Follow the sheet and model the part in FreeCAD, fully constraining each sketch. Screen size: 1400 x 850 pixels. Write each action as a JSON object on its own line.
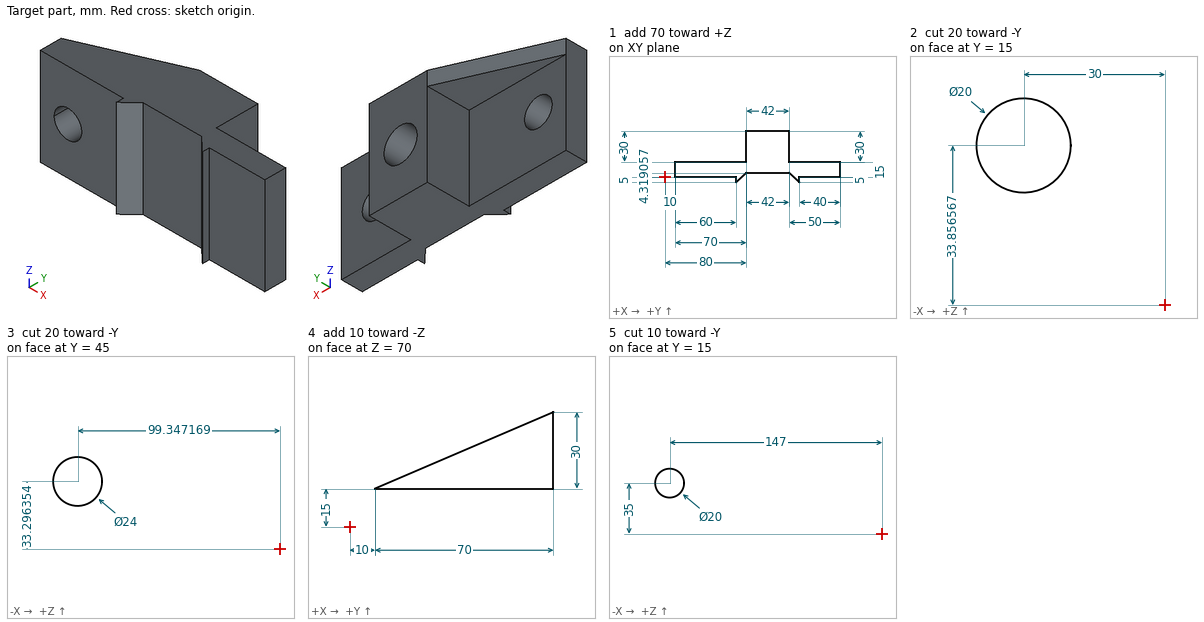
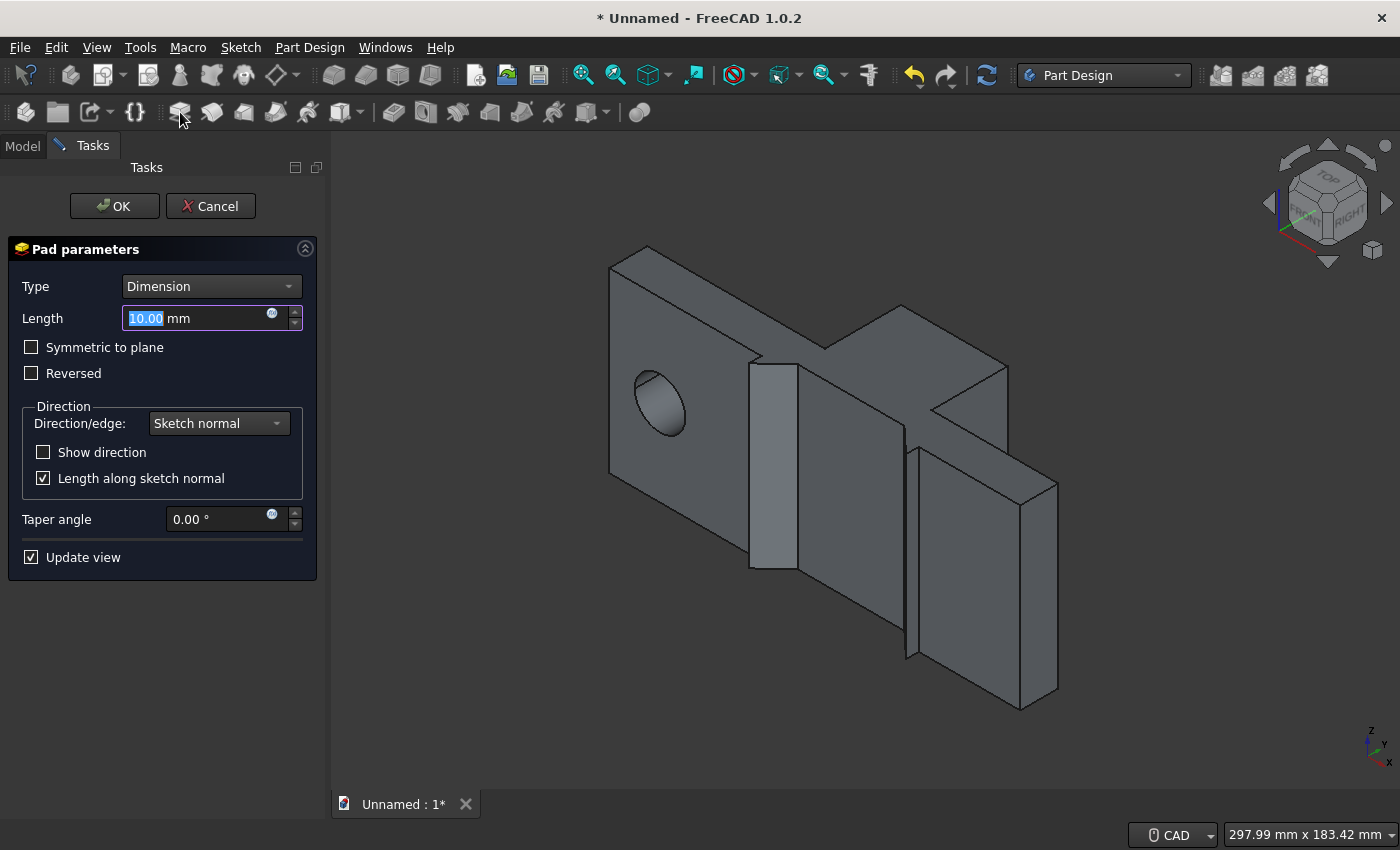
{"action": "type", "text": "10"}
{"action": "key", "text": "Tab"}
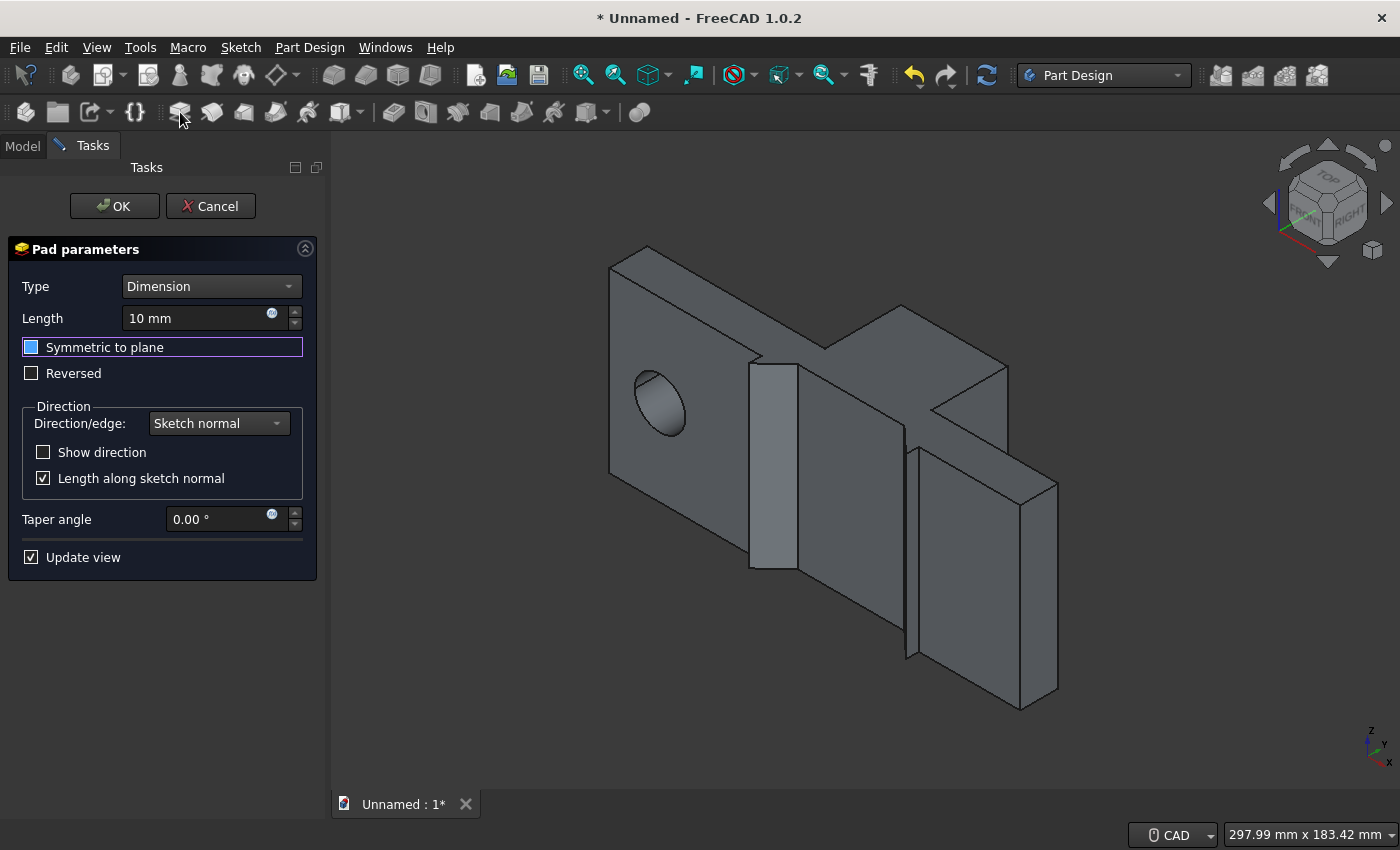
{"action": "left_click", "coordinate": [30, 373]}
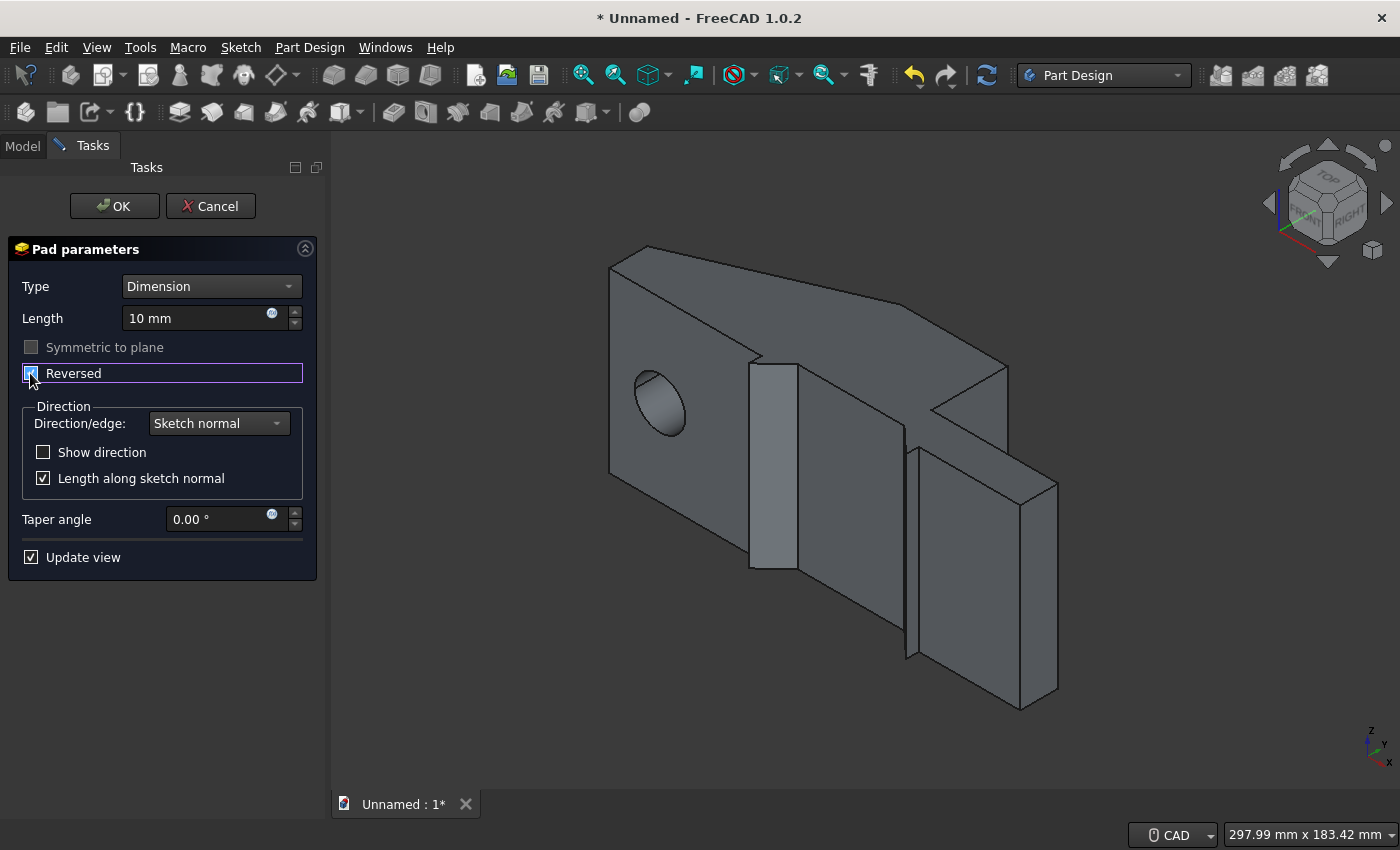
{"action": "left_click", "coordinate": [115, 206]}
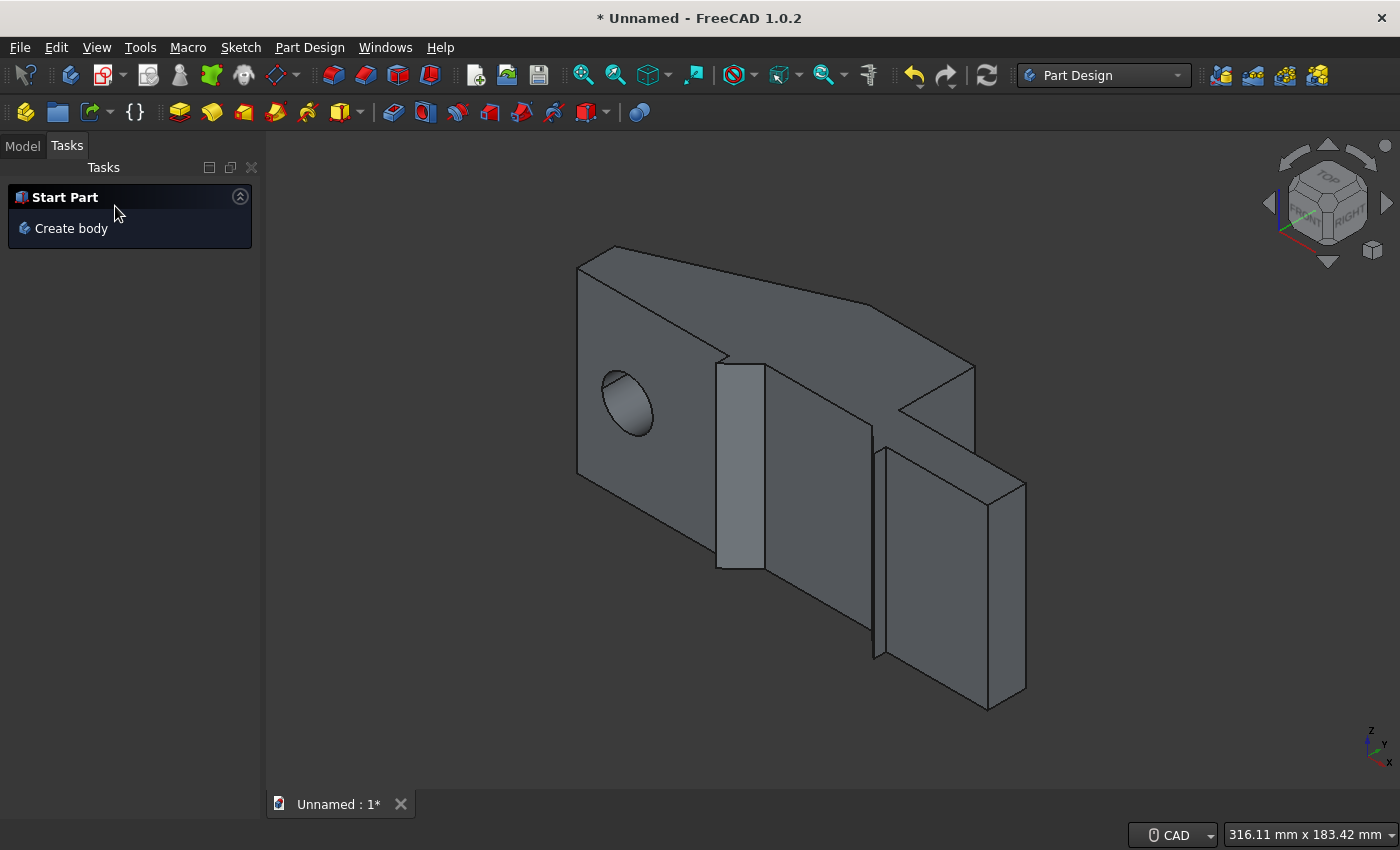
{"action": "key", "text": "4"}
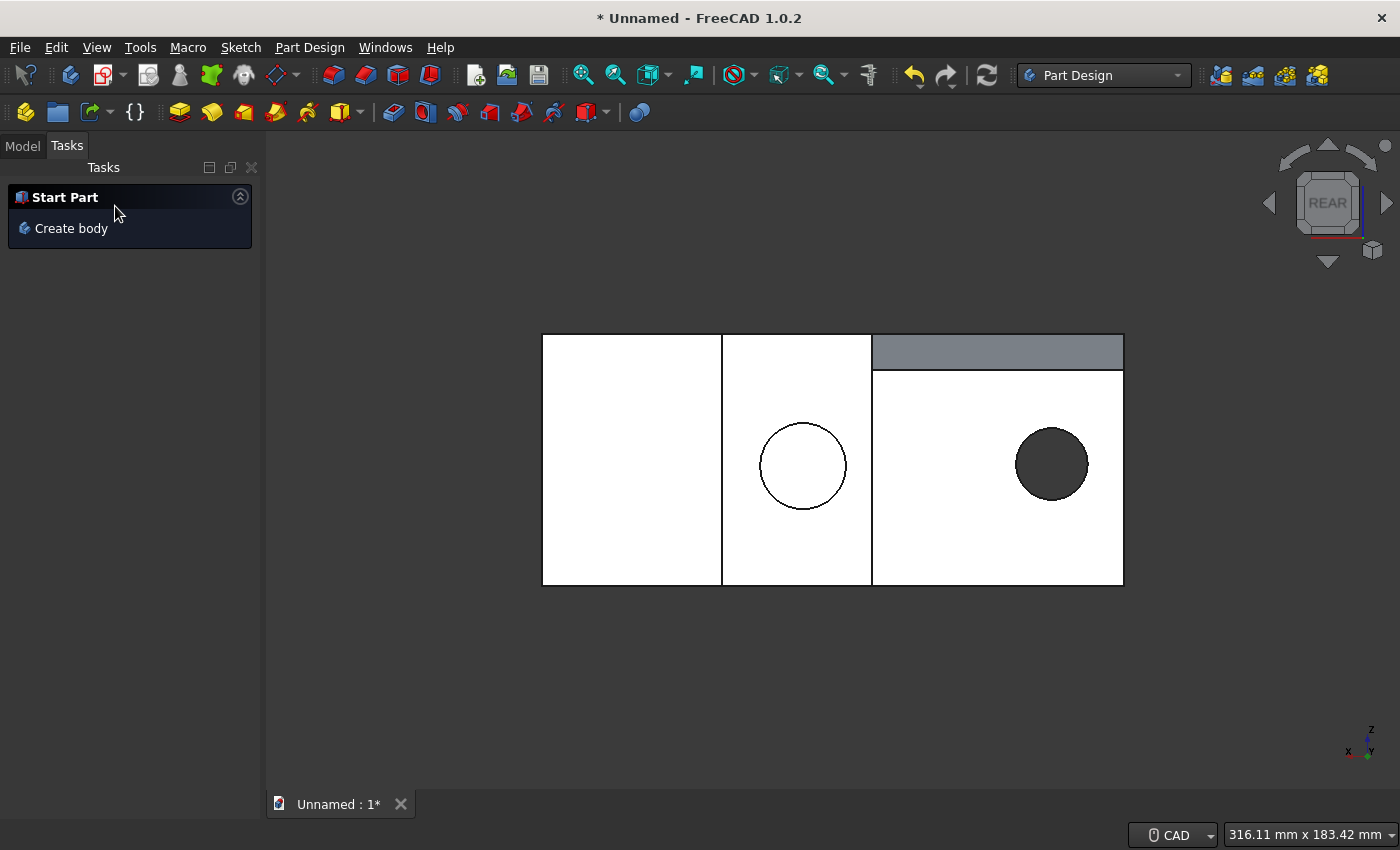
{"action": "left_click", "coordinate": [962, 508]}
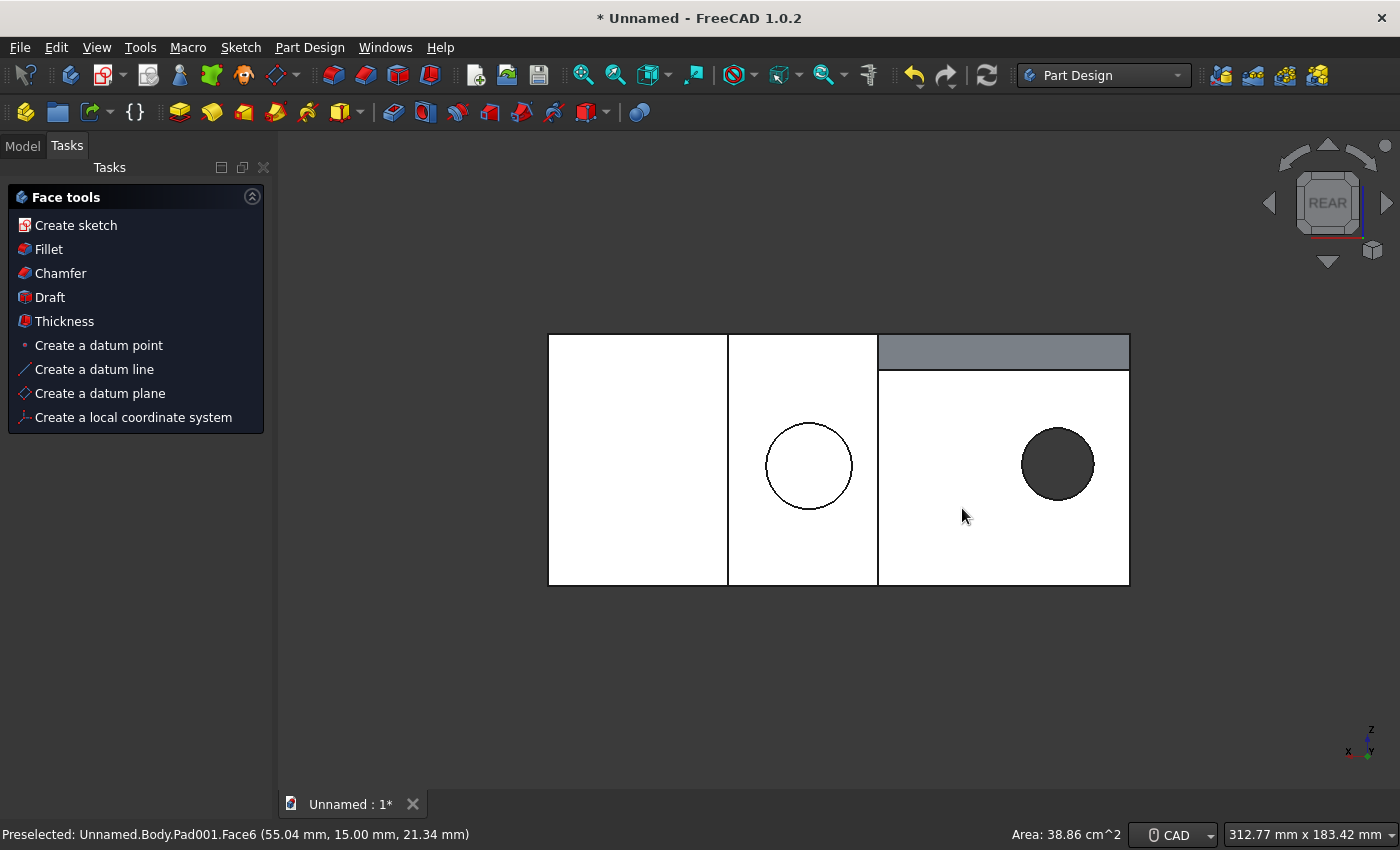
{"action": "left_click", "coordinate": [104, 76]}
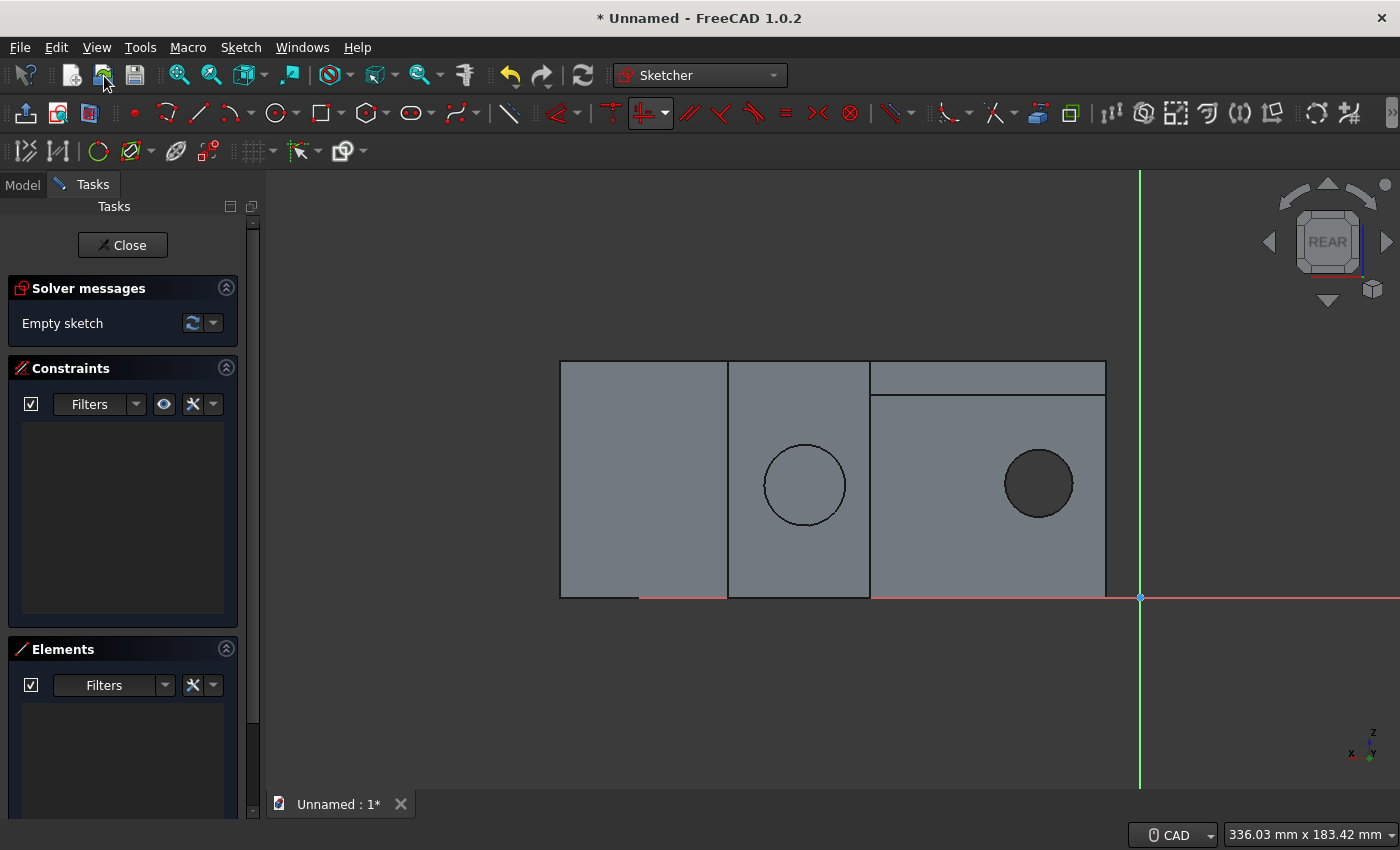
{"action": "scroll", "coordinate": [620, 480], "scroll_direction": "up", "scroll_amount": 9}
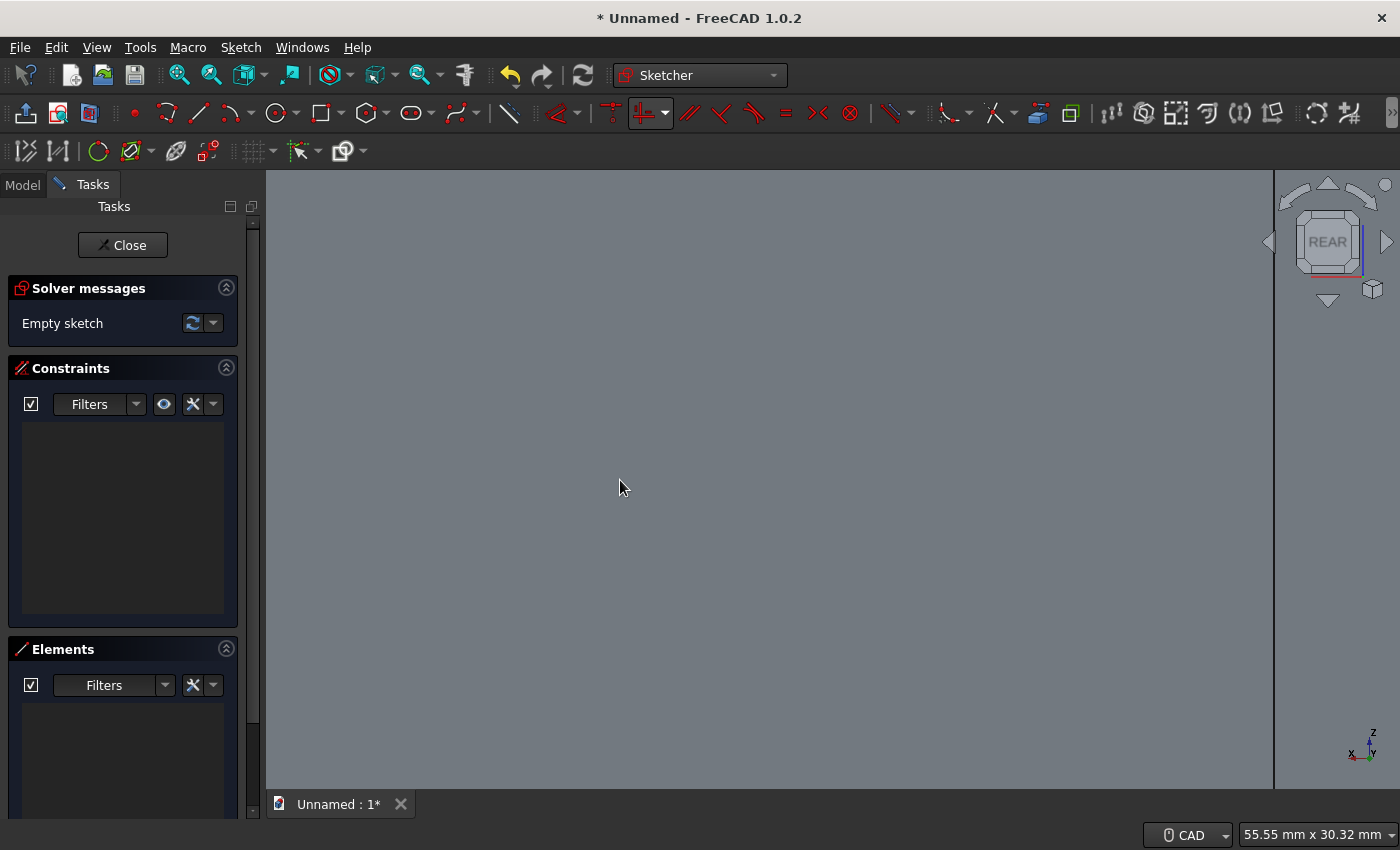
{"action": "left_click", "coordinate": [276, 114]}